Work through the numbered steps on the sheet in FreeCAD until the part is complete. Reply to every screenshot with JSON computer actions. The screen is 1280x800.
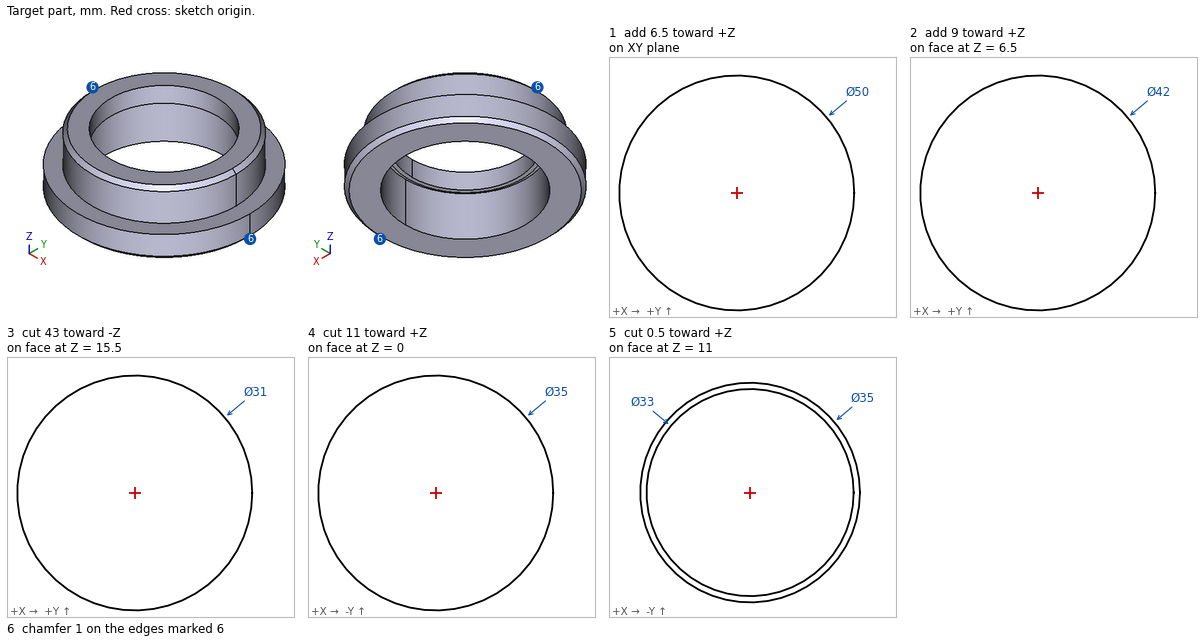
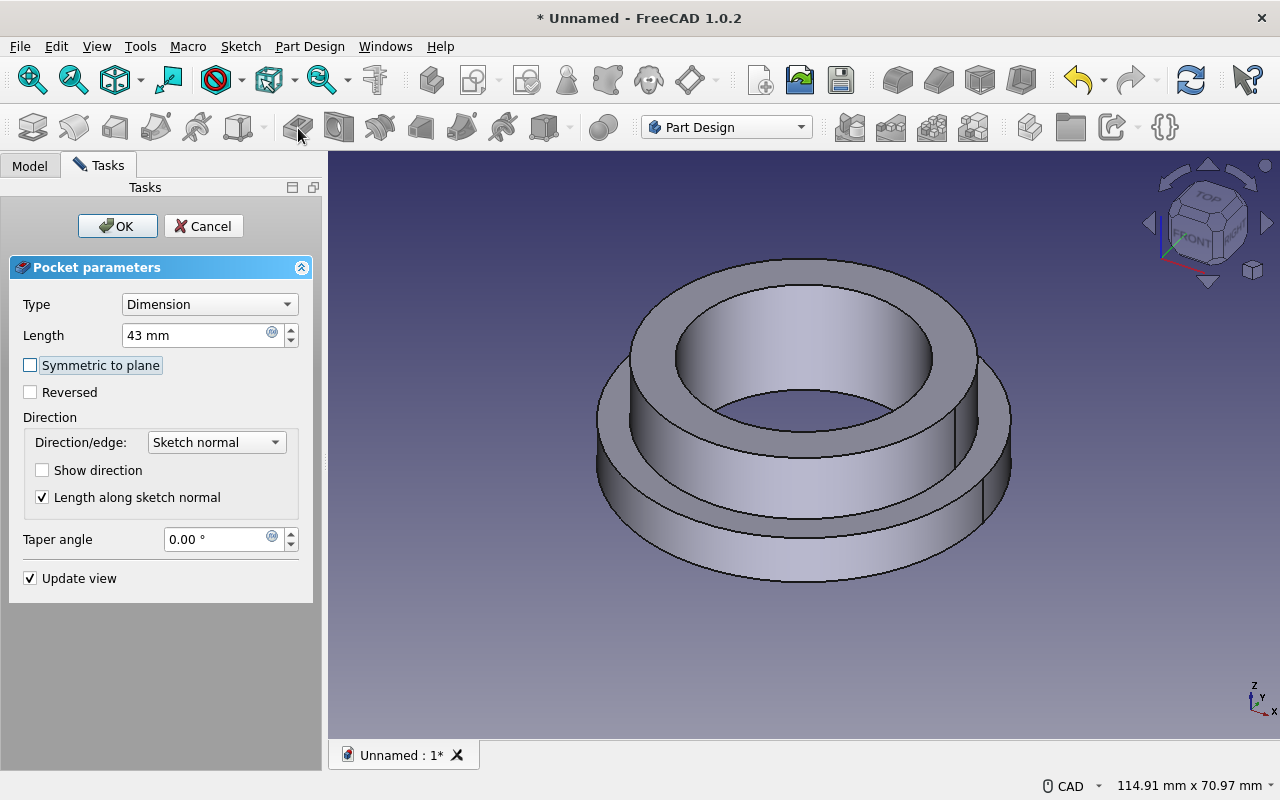
{"action": "left_click", "coordinate": [118, 226]}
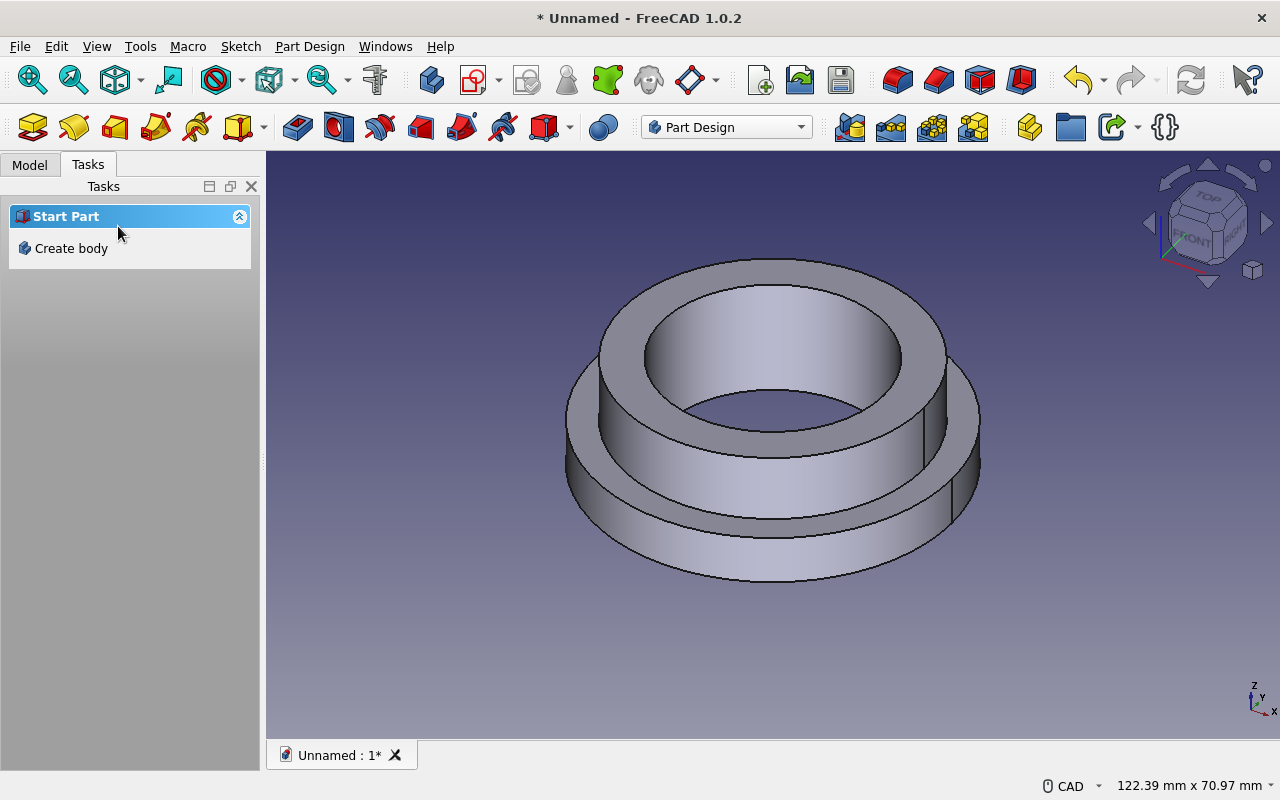
{"action": "key", "text": "5"}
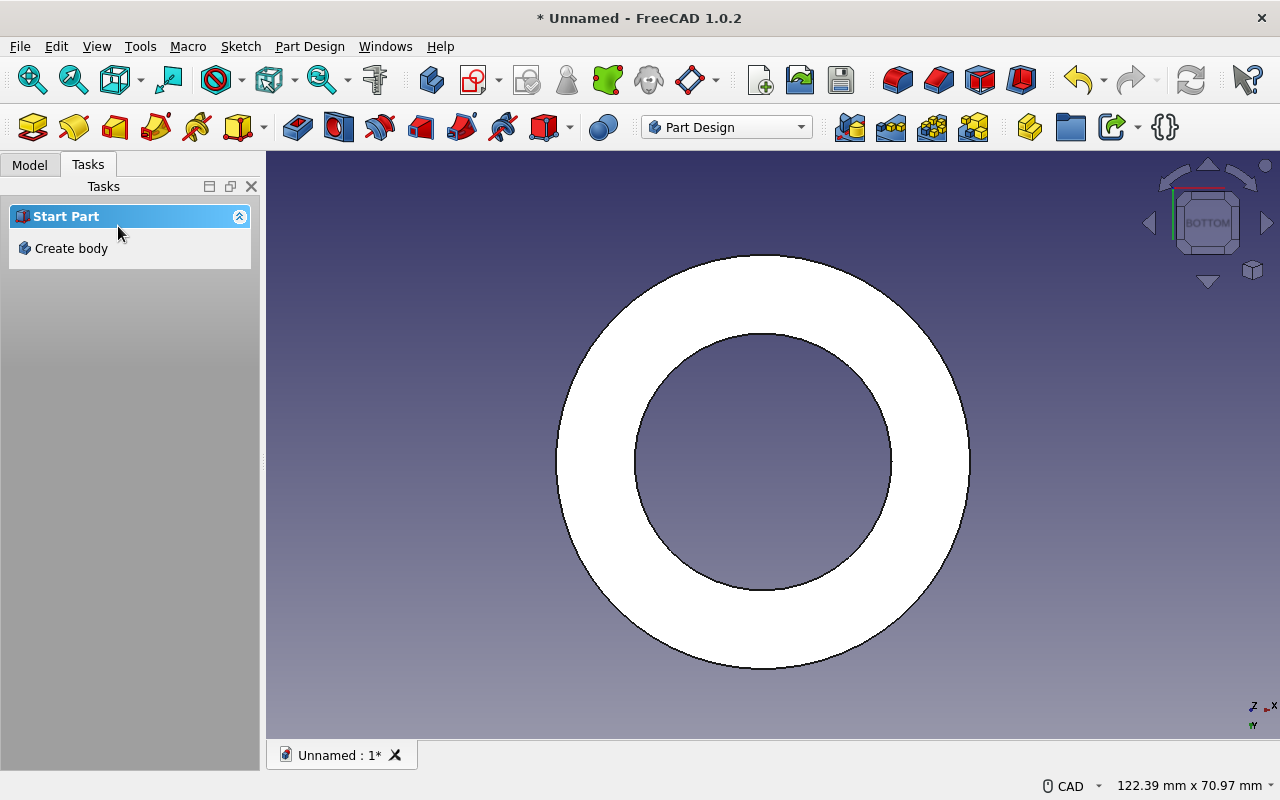
{"action": "left_click", "coordinate": [645, 579]}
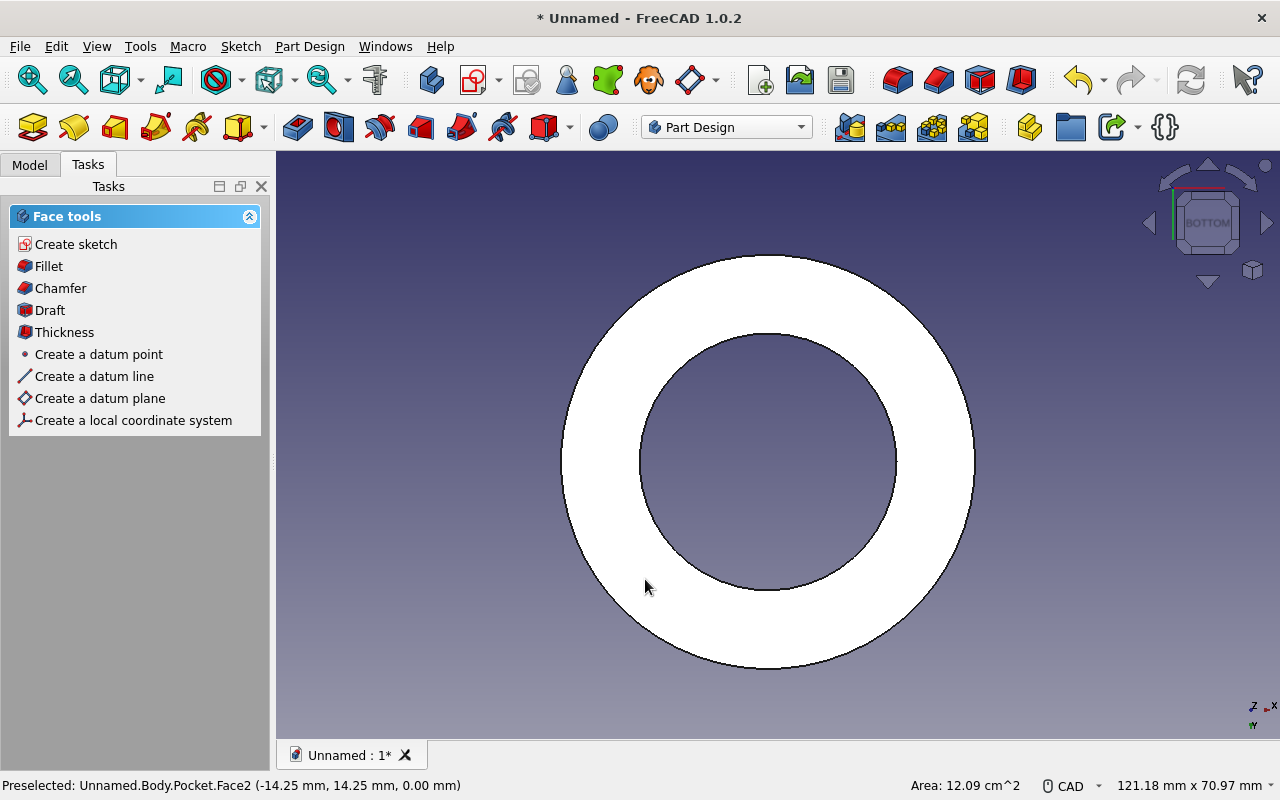
{"action": "left_click", "coordinate": [472, 80]}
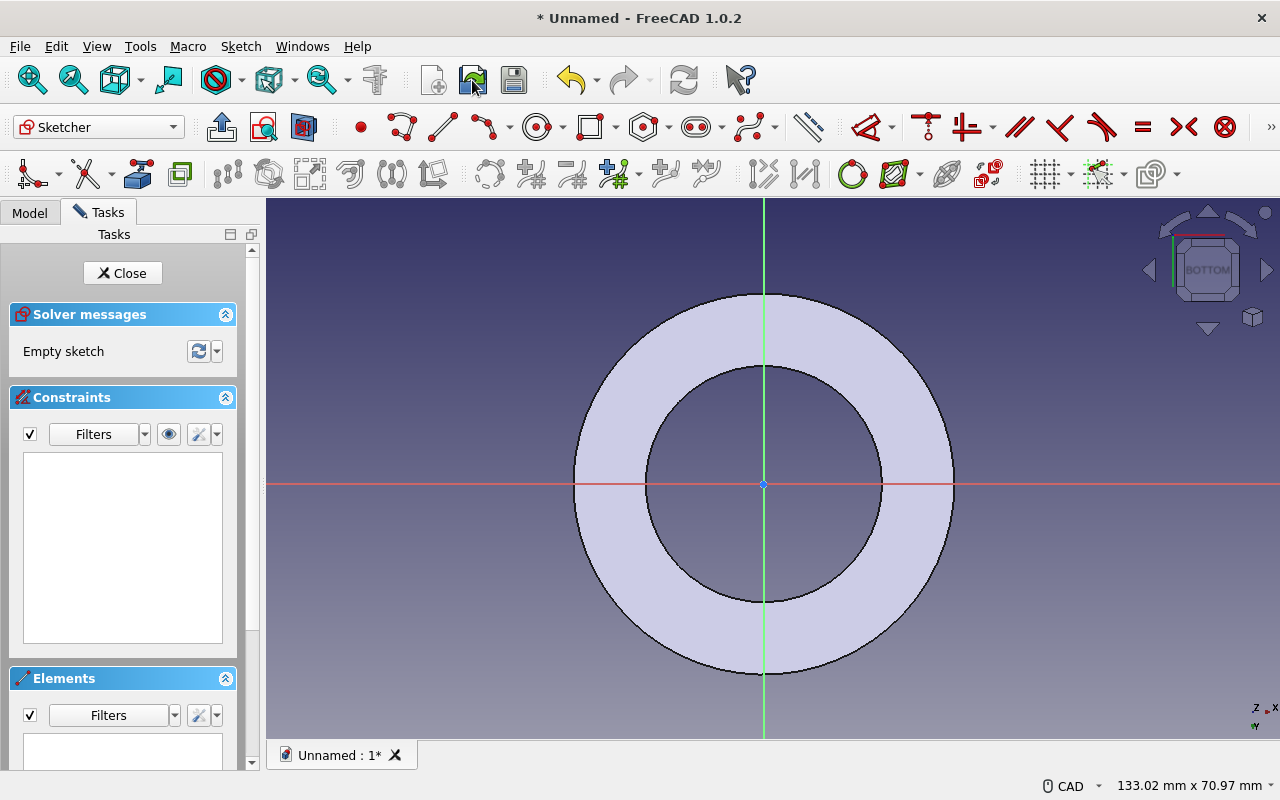
{"action": "left_click", "coordinate": [536, 128]}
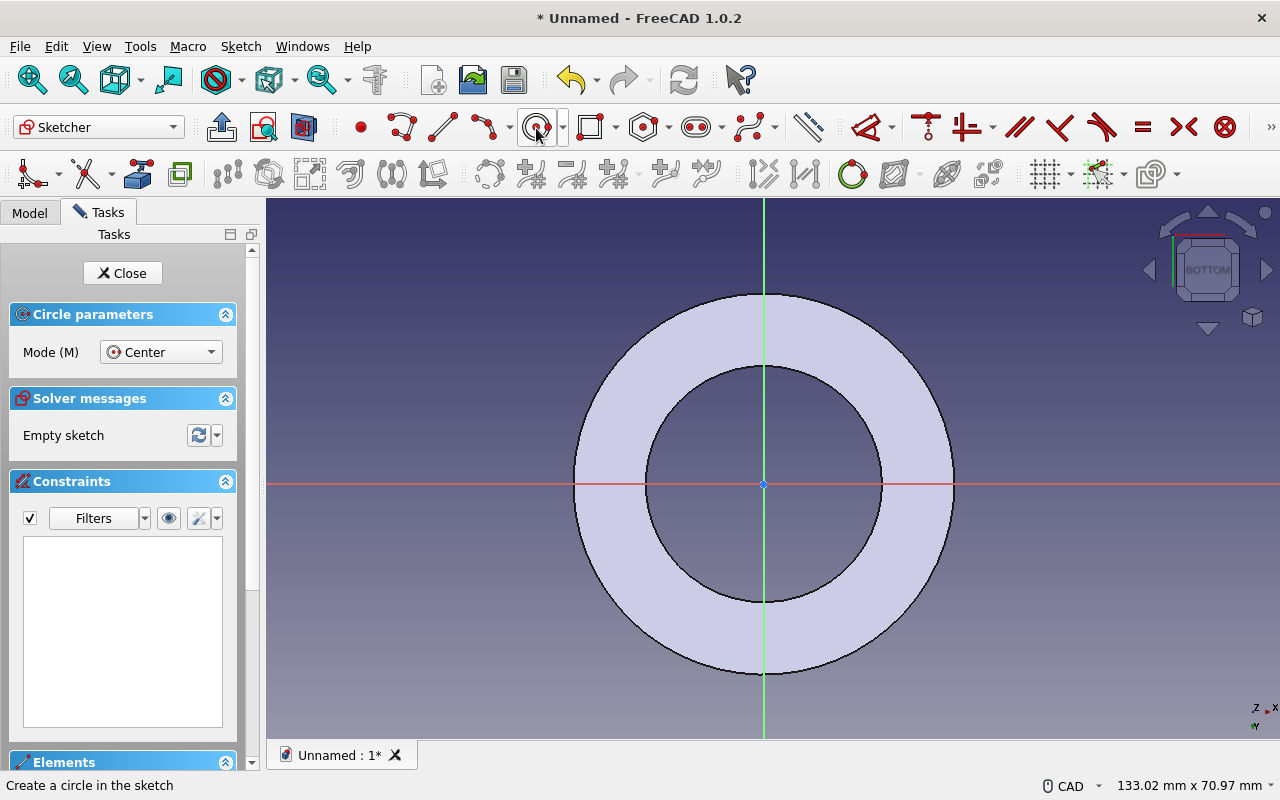
{"action": "left_click", "coordinate": [764, 484]}
{"action": "mouse_move", "coordinate": [858, 390]}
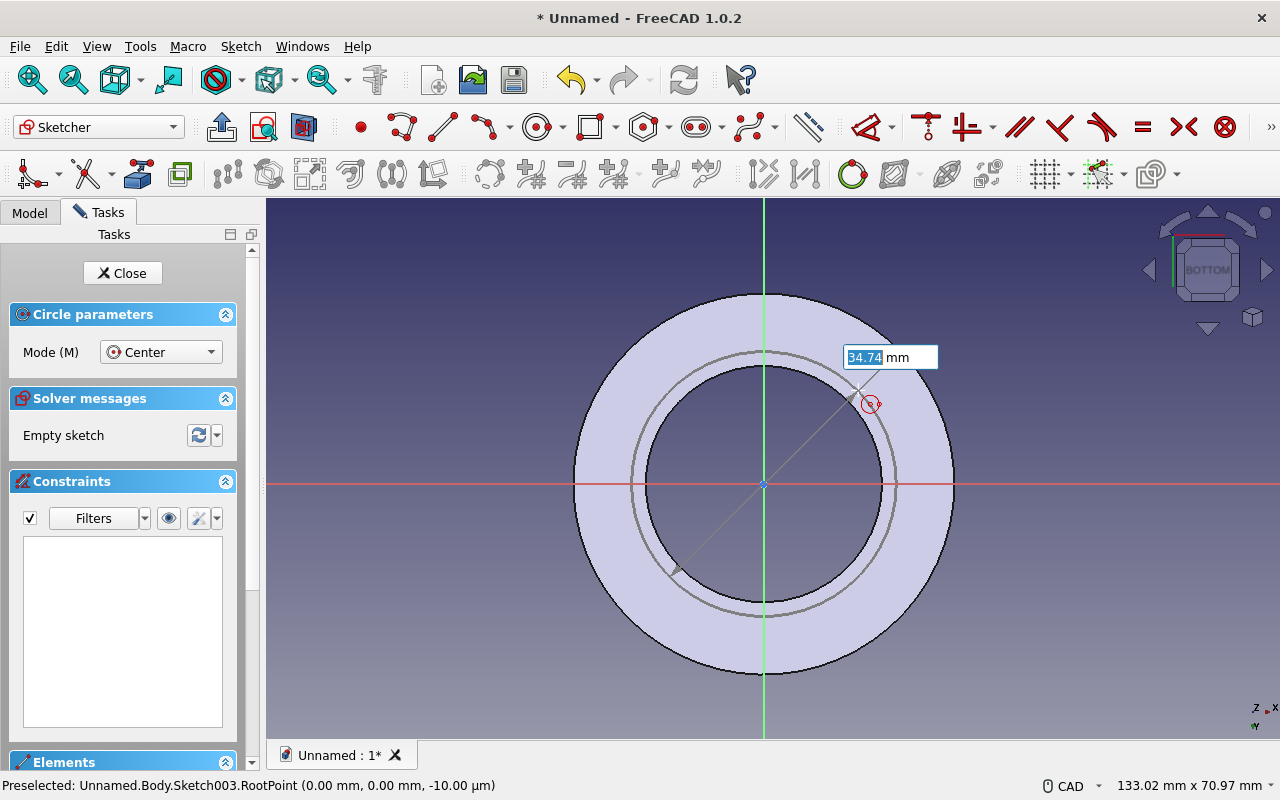
{"action": "type", "text": "35"}
{"action": "key", "text": "Return"}
{"action": "key", "text": "Escape"}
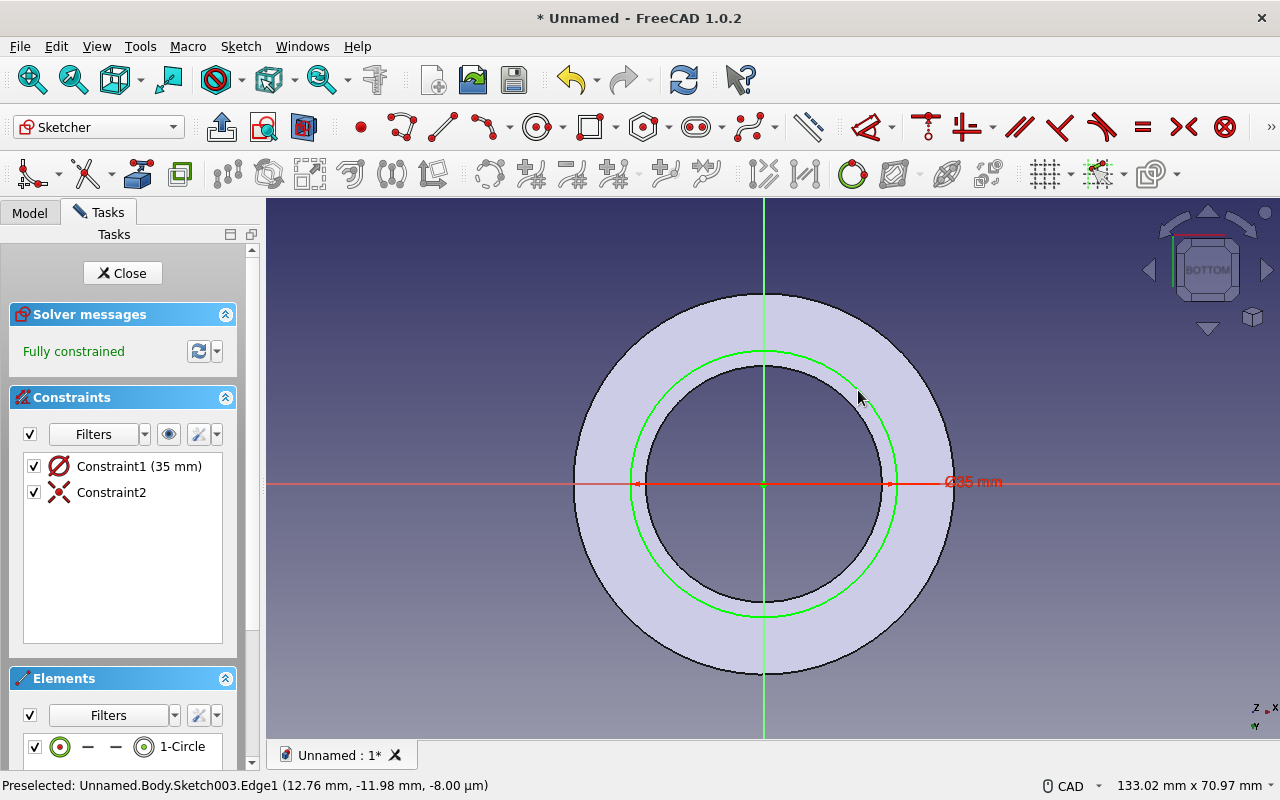
{"action": "left_click", "coordinate": [123, 273]}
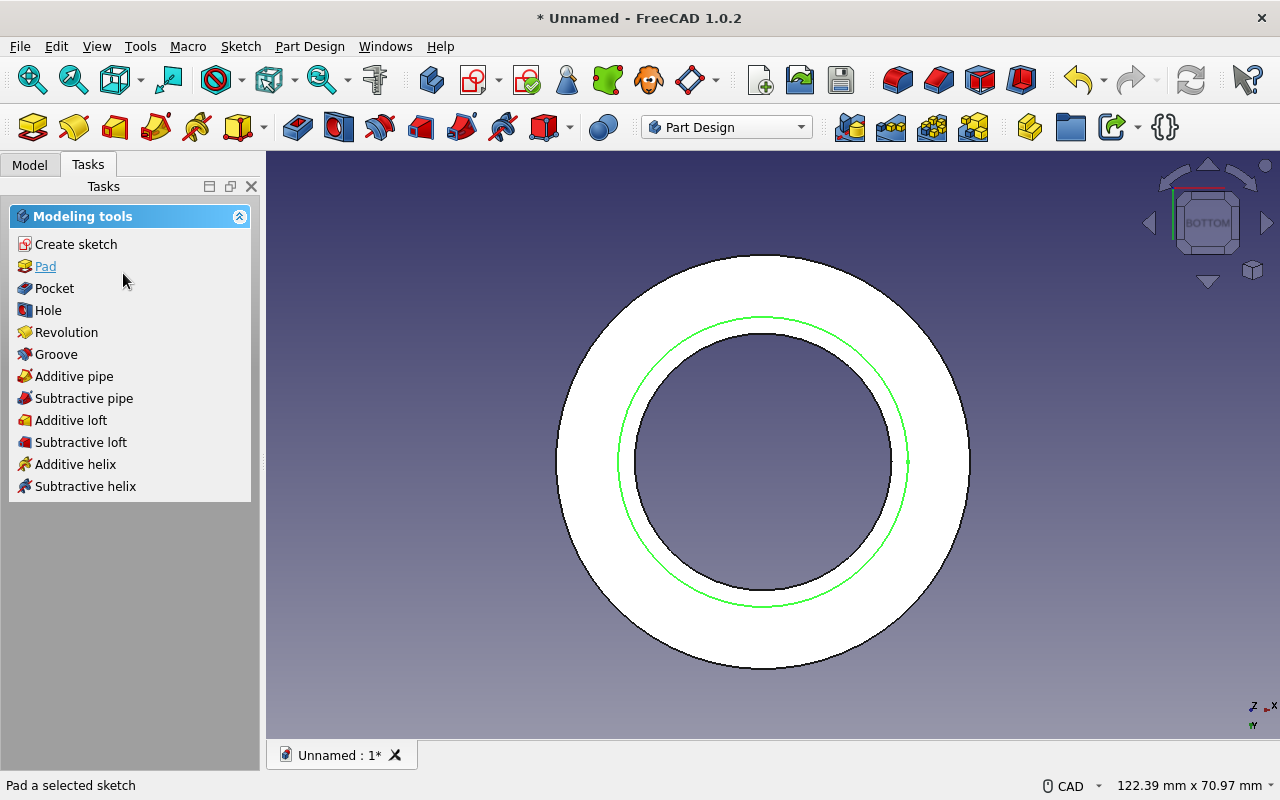
{"action": "left_click", "coordinate": [298, 128]}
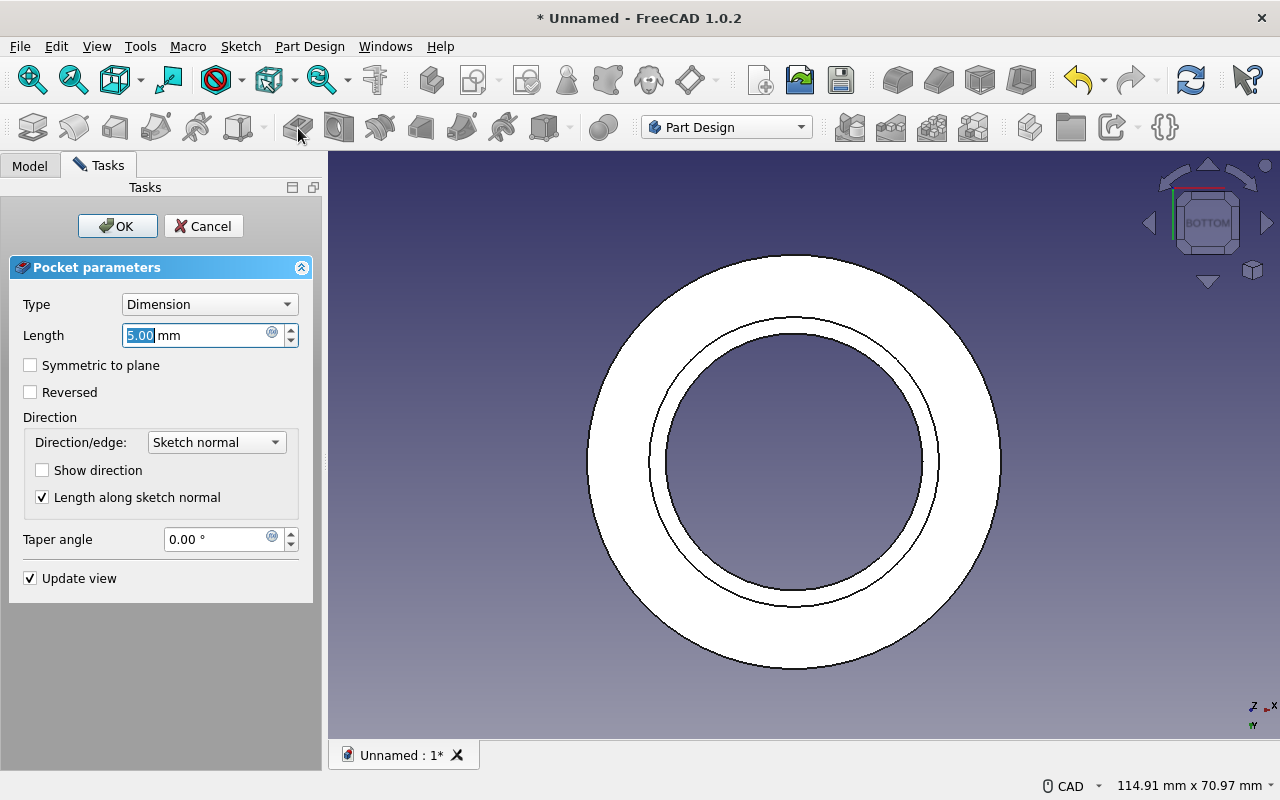
{"action": "type", "text": "11"}
{"action": "key", "text": "Tab"}